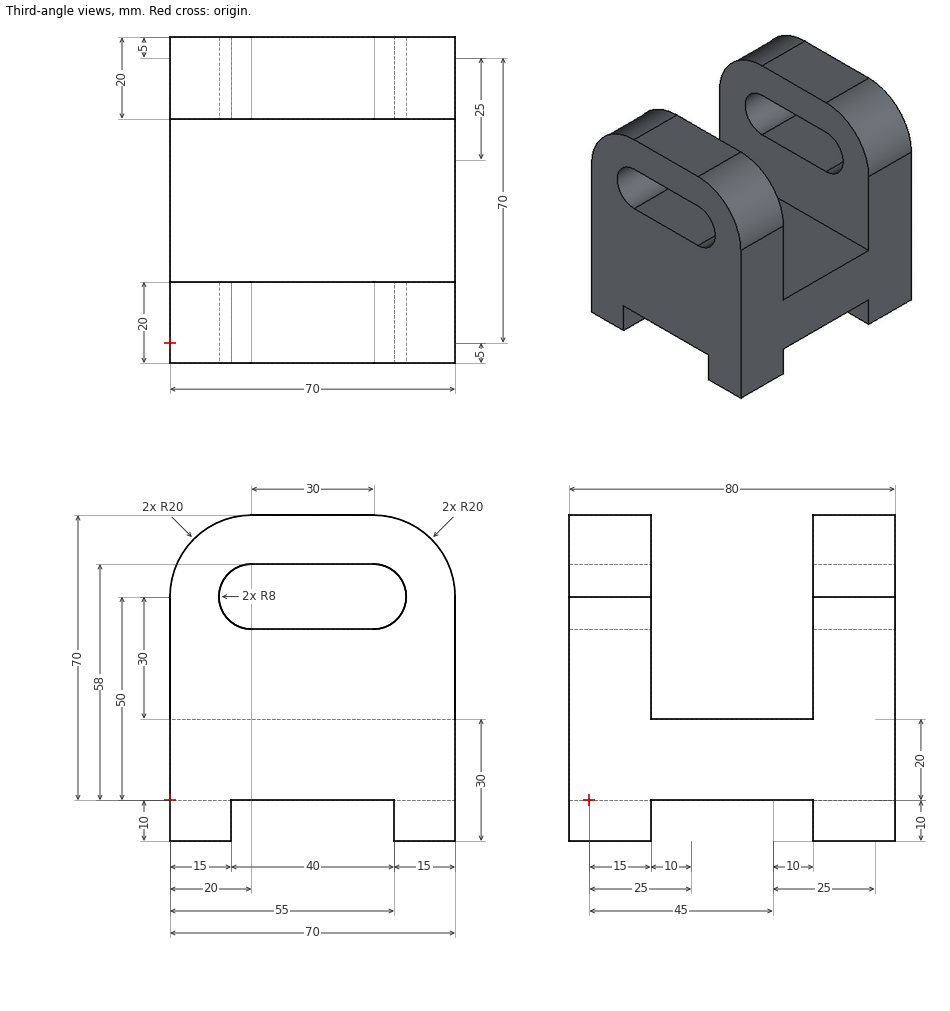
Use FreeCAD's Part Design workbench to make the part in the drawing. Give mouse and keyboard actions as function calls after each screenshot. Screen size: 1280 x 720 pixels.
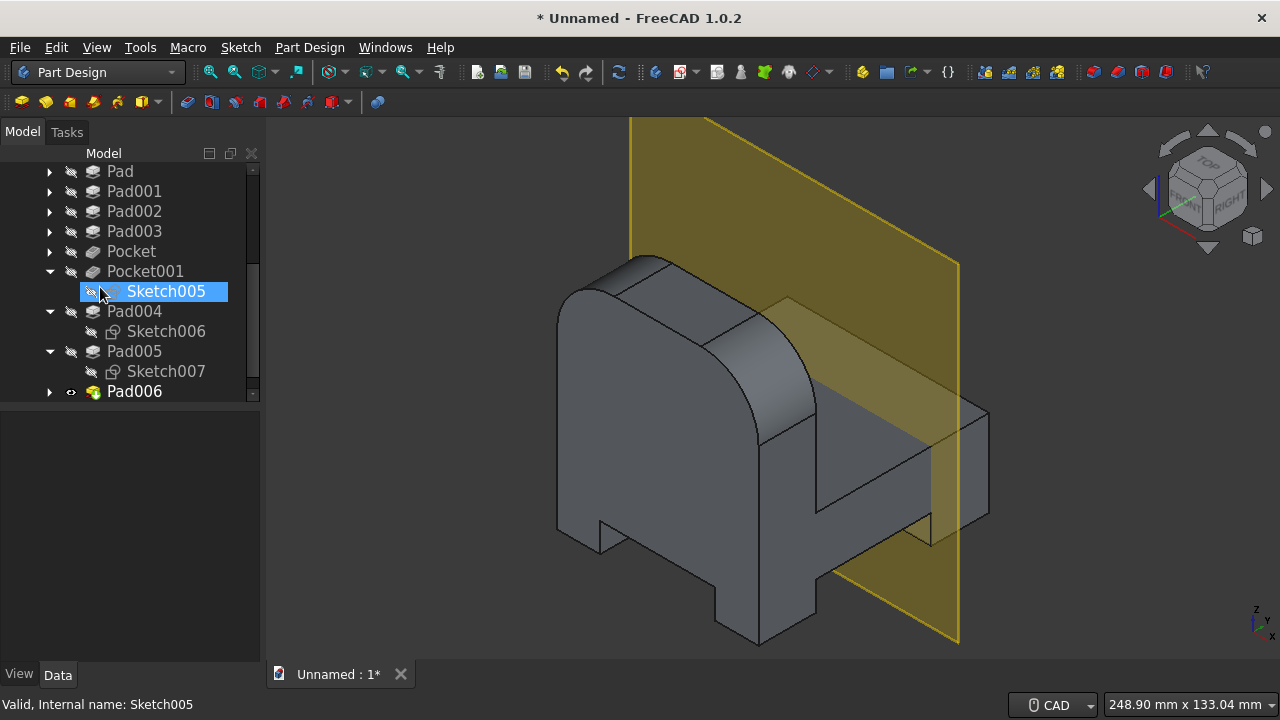
scroll(140, 287, up, 15)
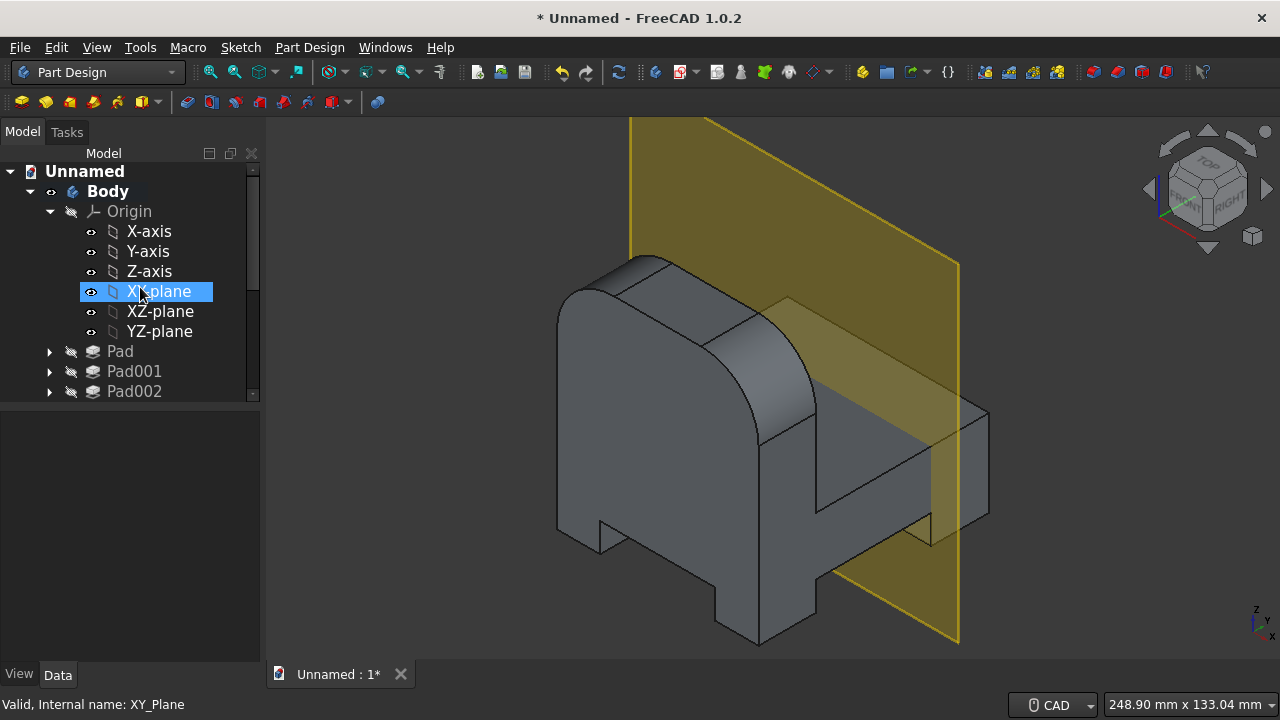
scroll(100, 287, down, 6)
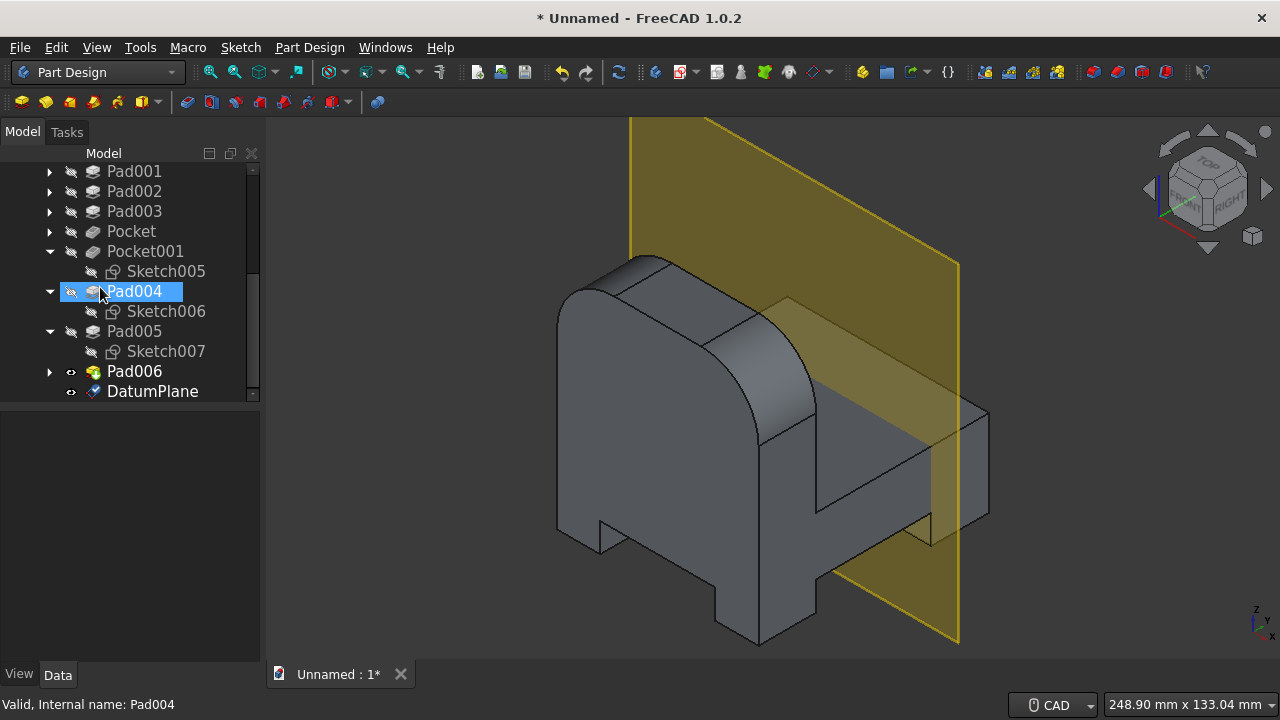
click(116, 392)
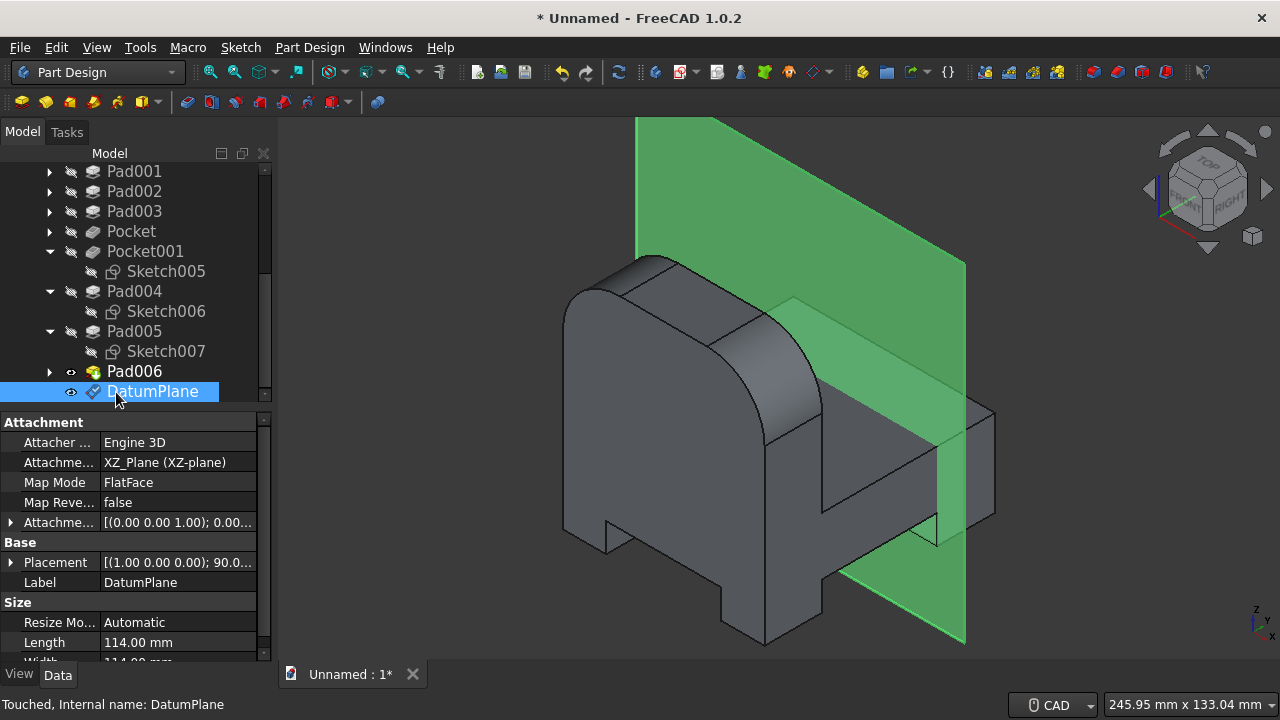
click(680, 72)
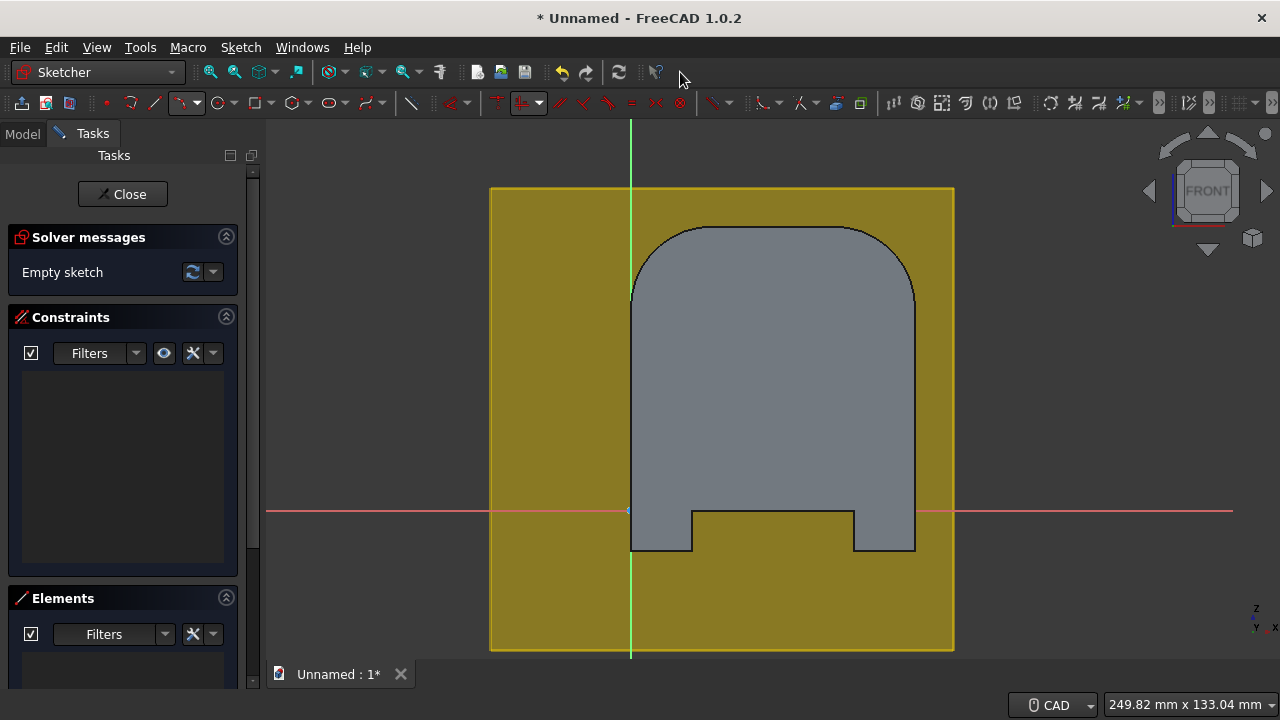
key(q)
key(s)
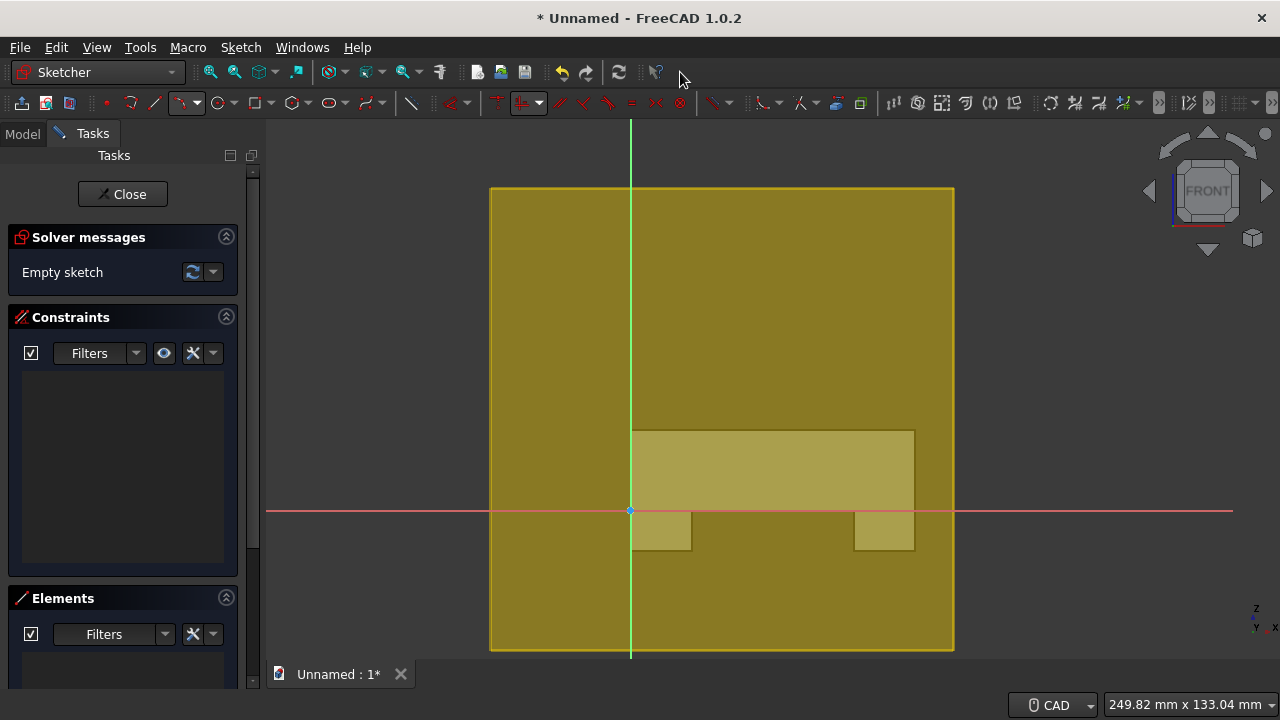
key(g)
key(l)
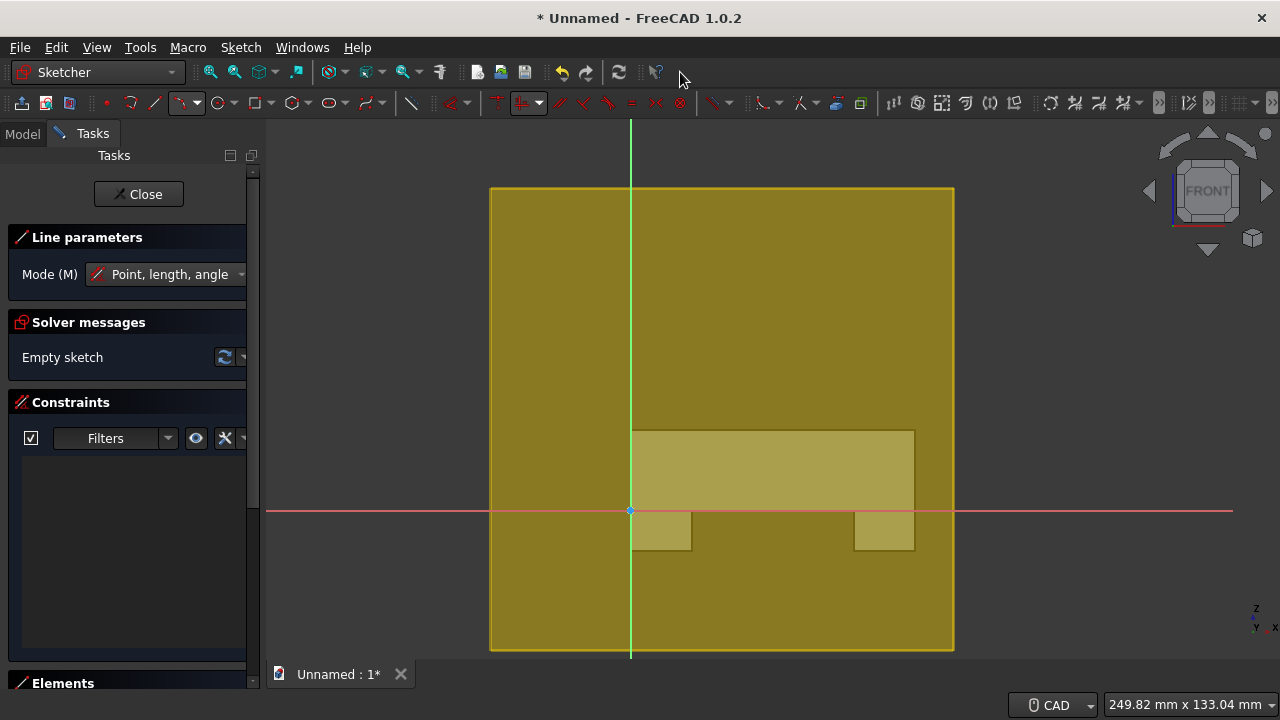
click(712, 227)
click(834, 227)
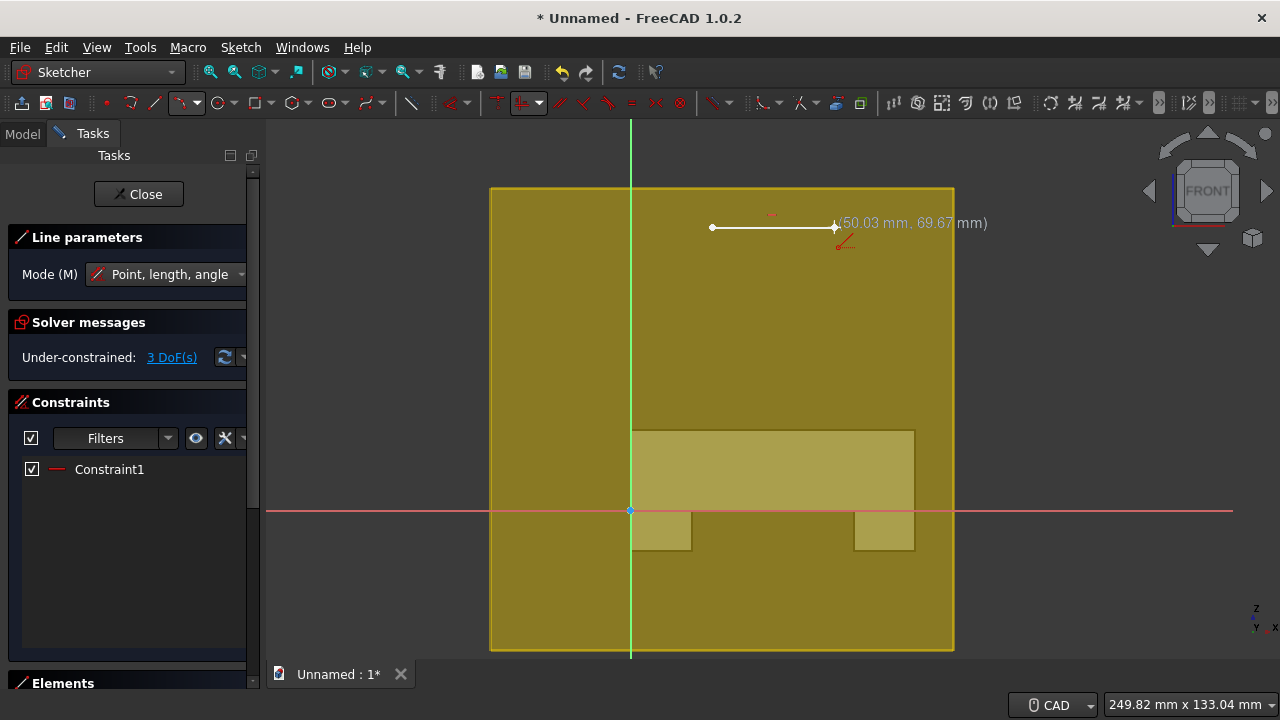
click(132, 104)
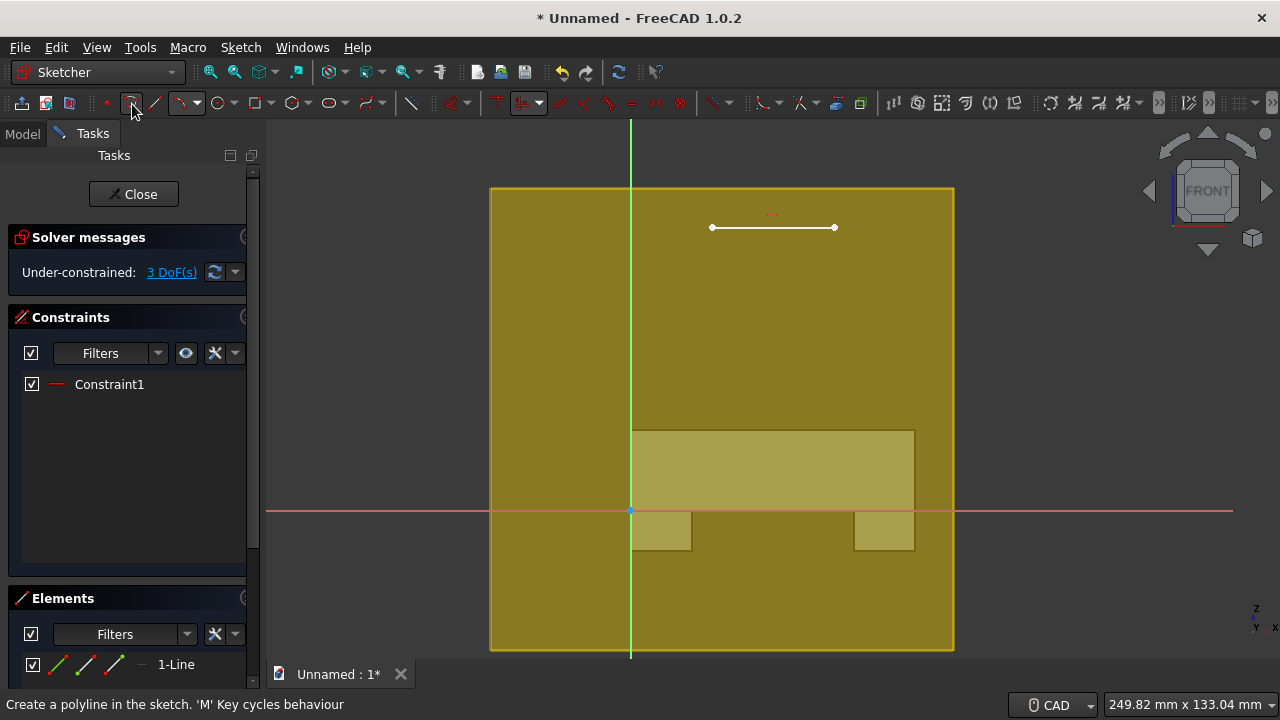
click(915, 308)
click(915, 430)
click(631, 430)
click(640, 308)
right_click(640, 308)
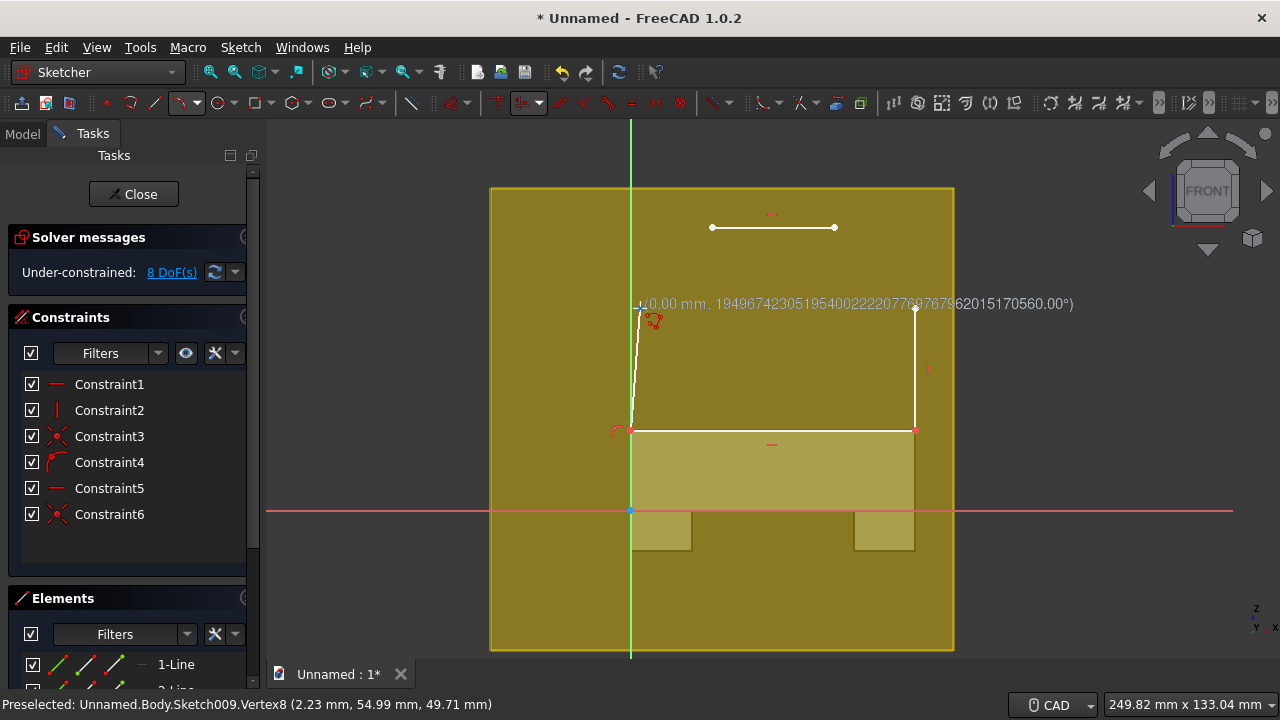
key(g)
key(3)
key(a)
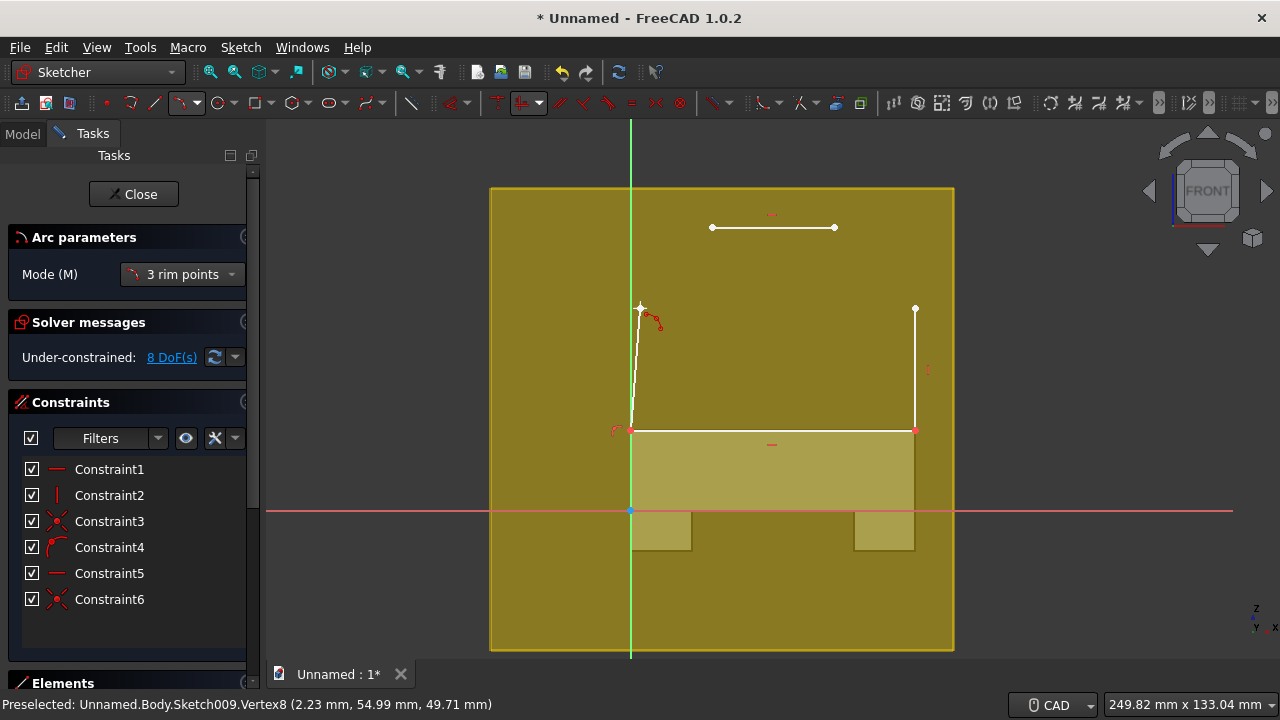
click(834, 228)
click(915, 309)
click(891, 250)